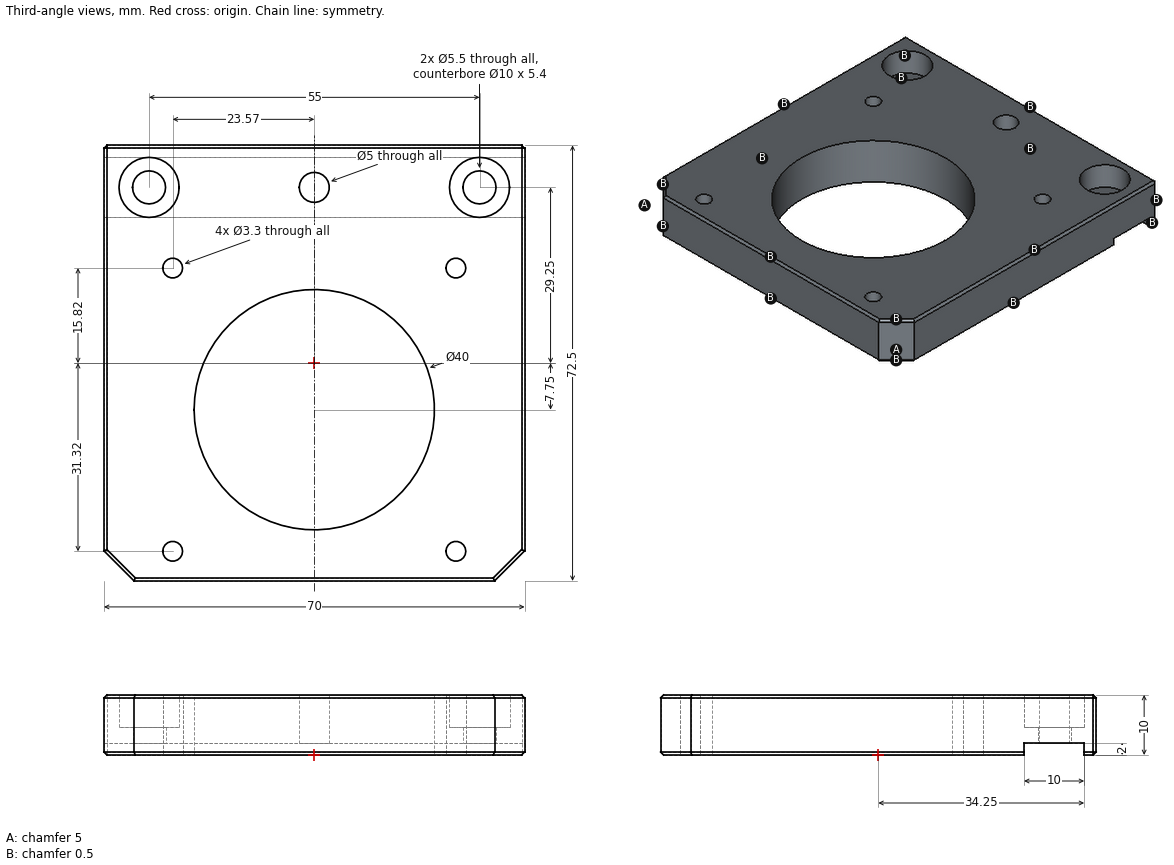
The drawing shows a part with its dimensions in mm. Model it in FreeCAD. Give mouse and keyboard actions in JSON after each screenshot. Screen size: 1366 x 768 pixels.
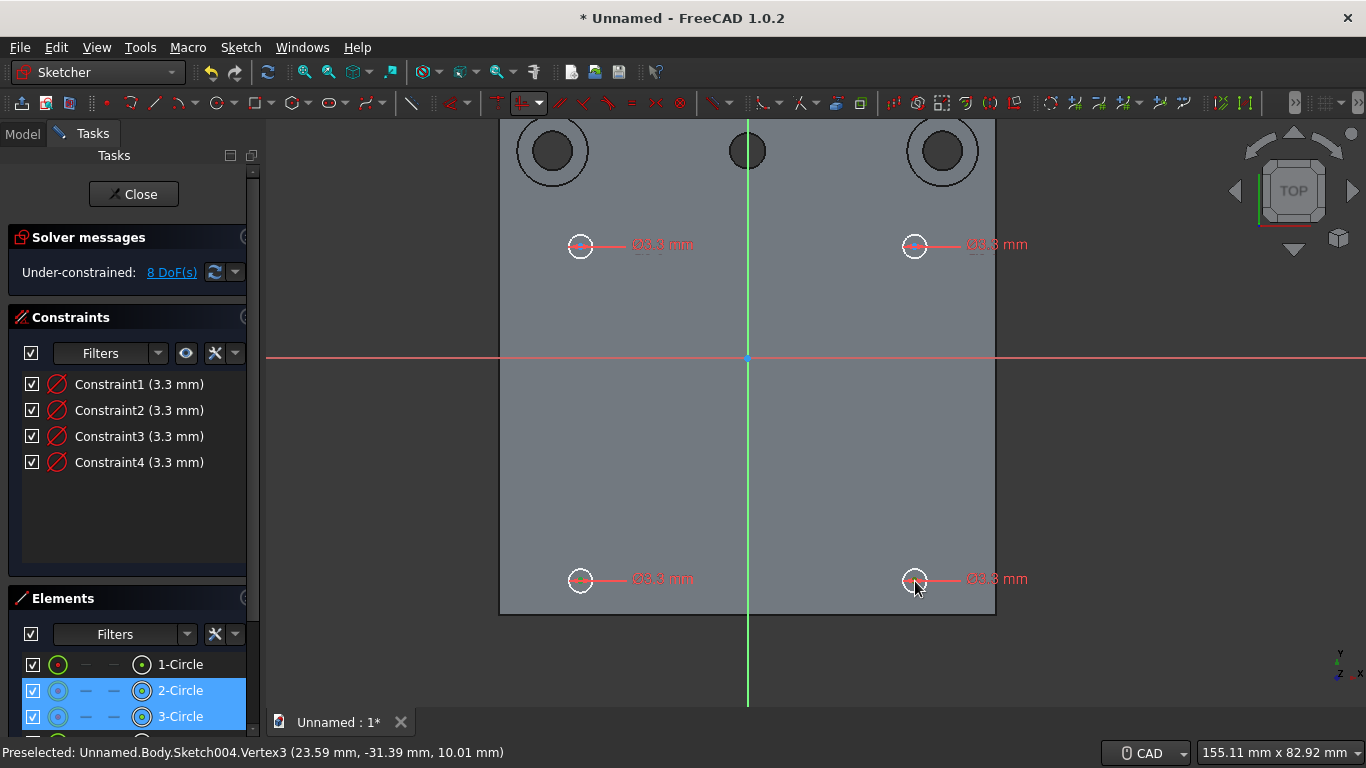
{"action": "left_click", "coordinate": [748, 641]}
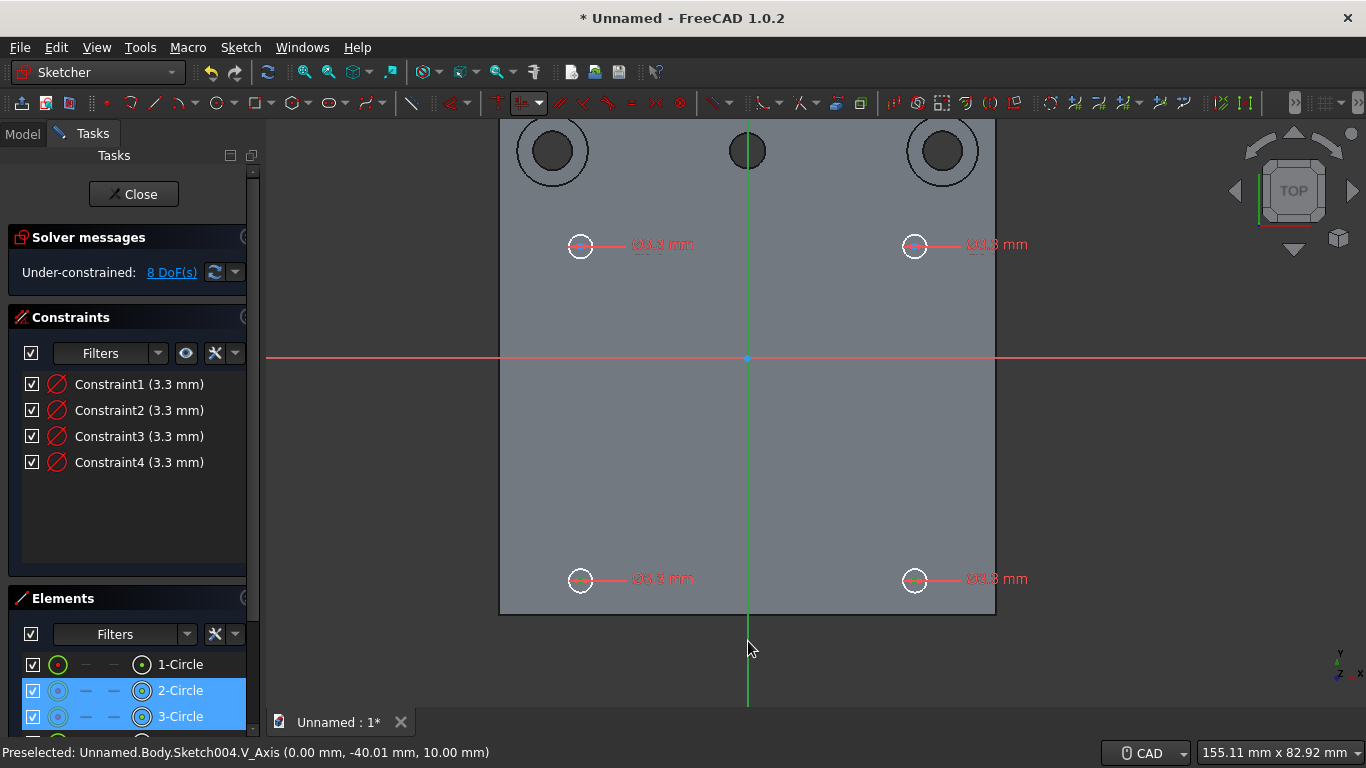
{"action": "left_click", "coordinate": [656, 104]}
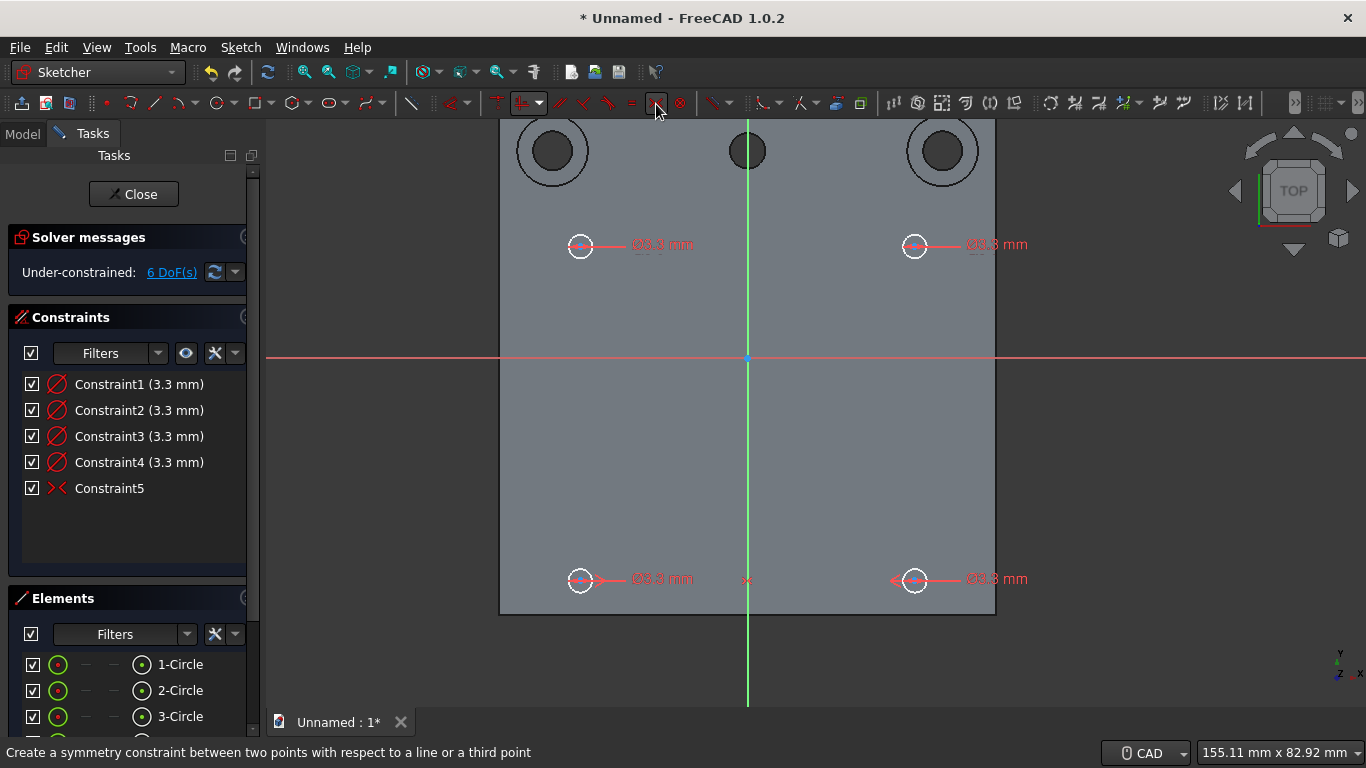
{"action": "left_click", "coordinate": [581, 247]}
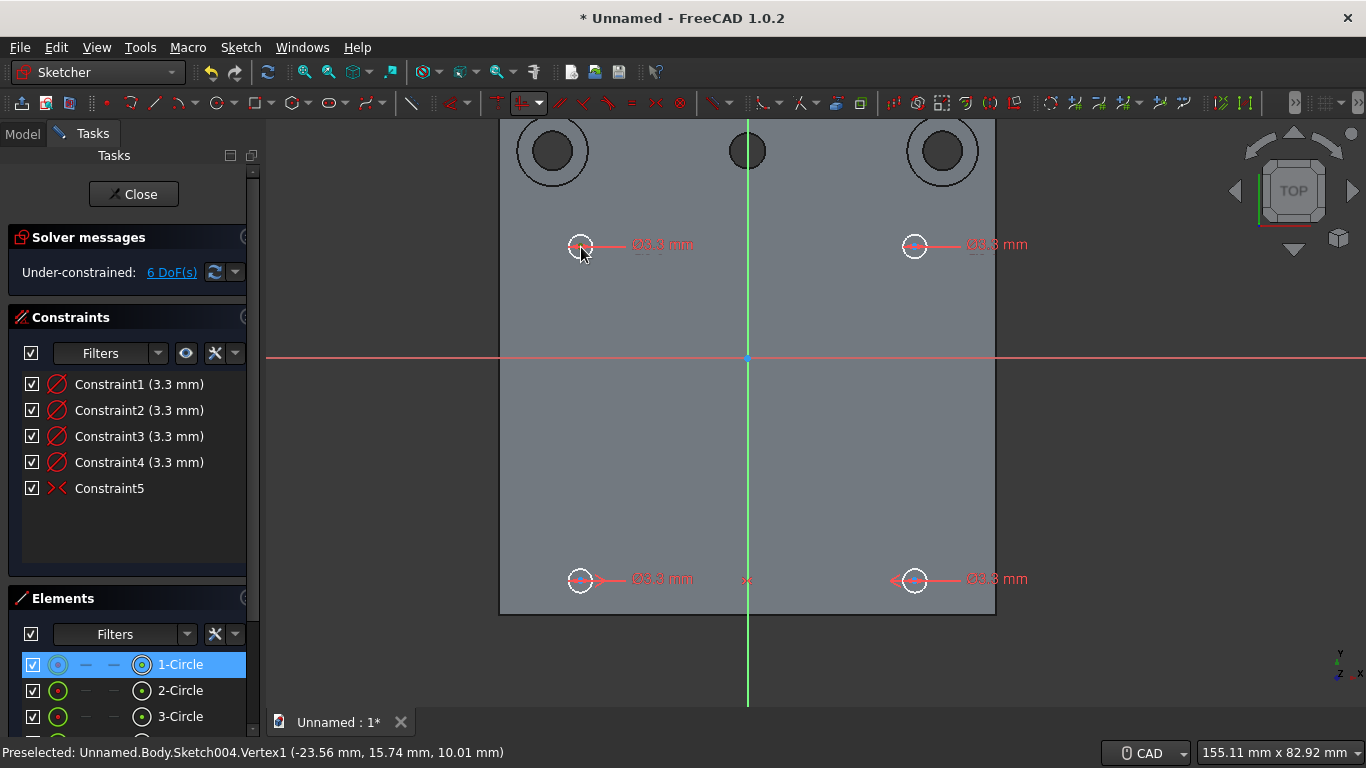
{"action": "left_click", "coordinate": [915, 247]}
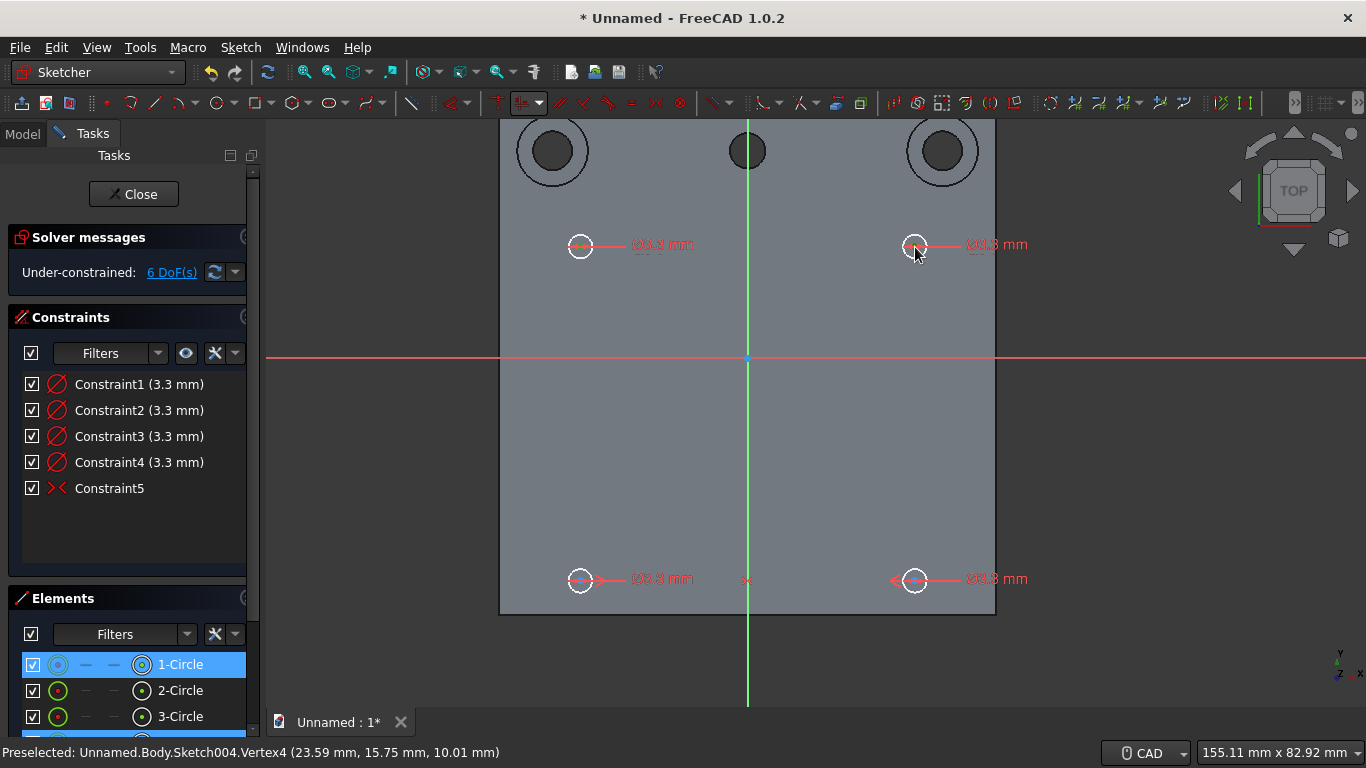
{"action": "left_click", "coordinate": [748, 641]}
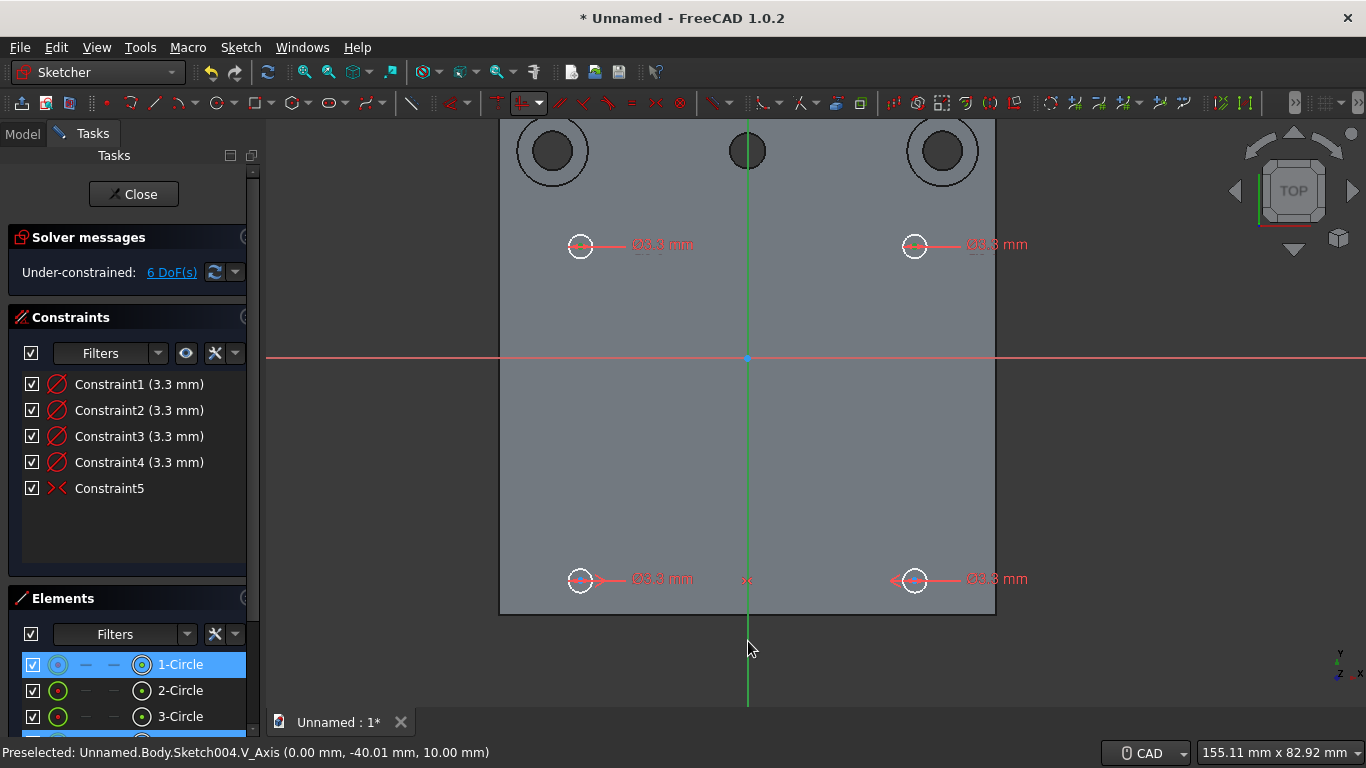
{"action": "left_click", "coordinate": [656, 104]}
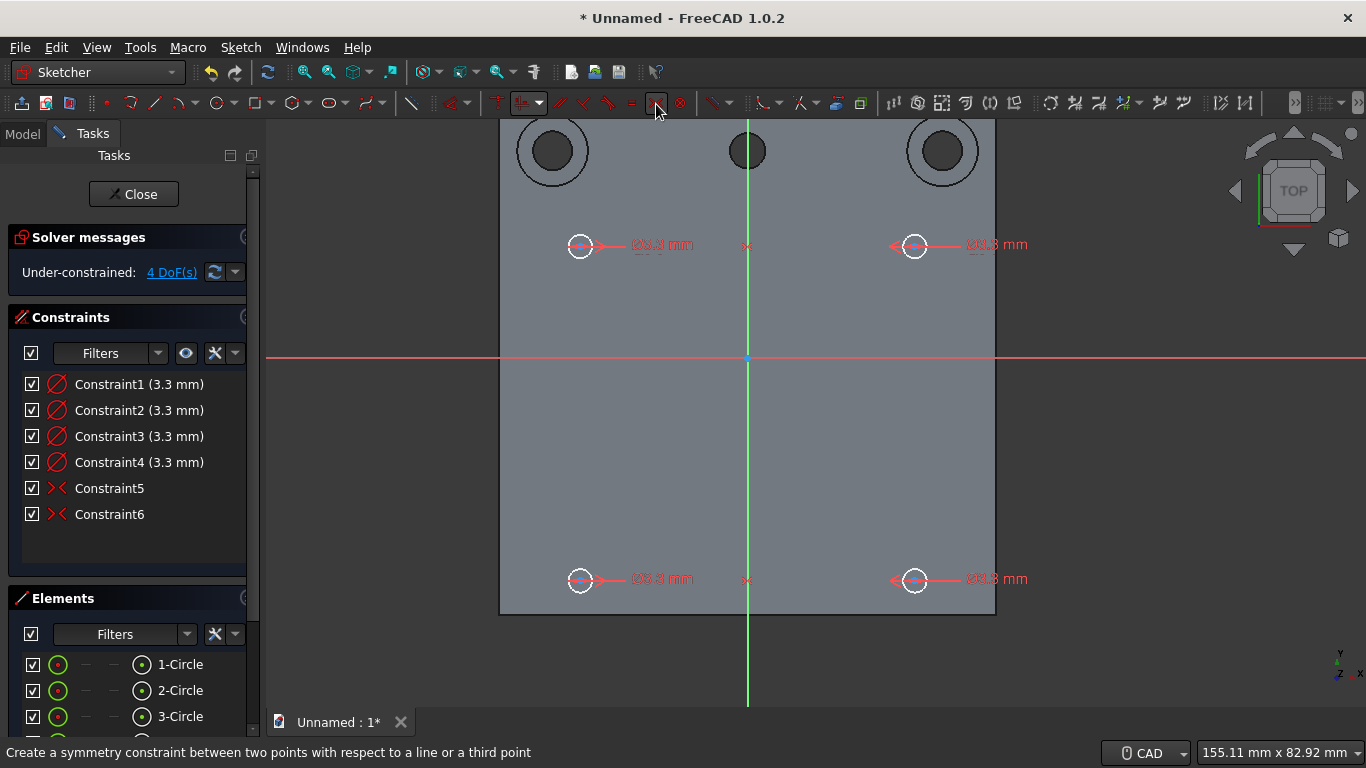
{"action": "left_click", "coordinate": [450, 104]}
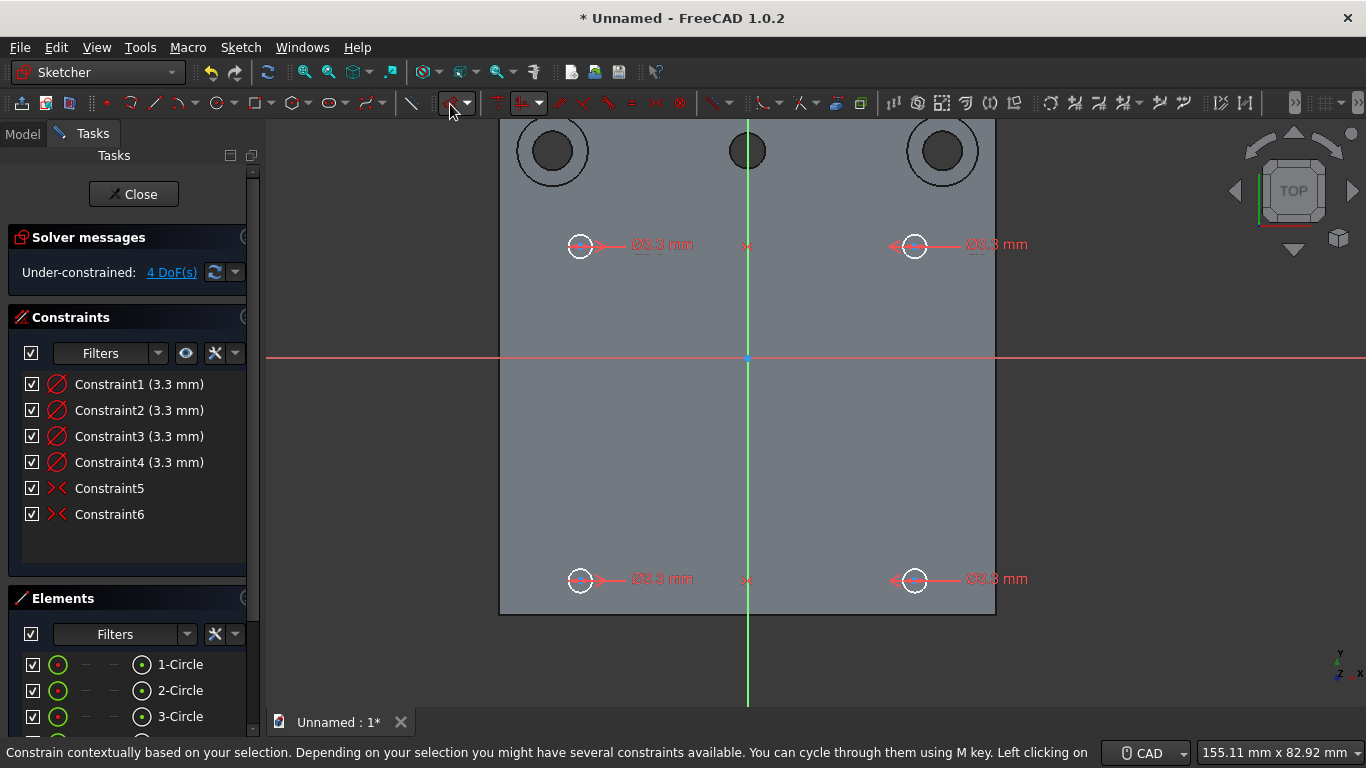
{"action": "left_click", "coordinate": [580, 247]}
{"action": "left_click", "coordinate": [664, 213]}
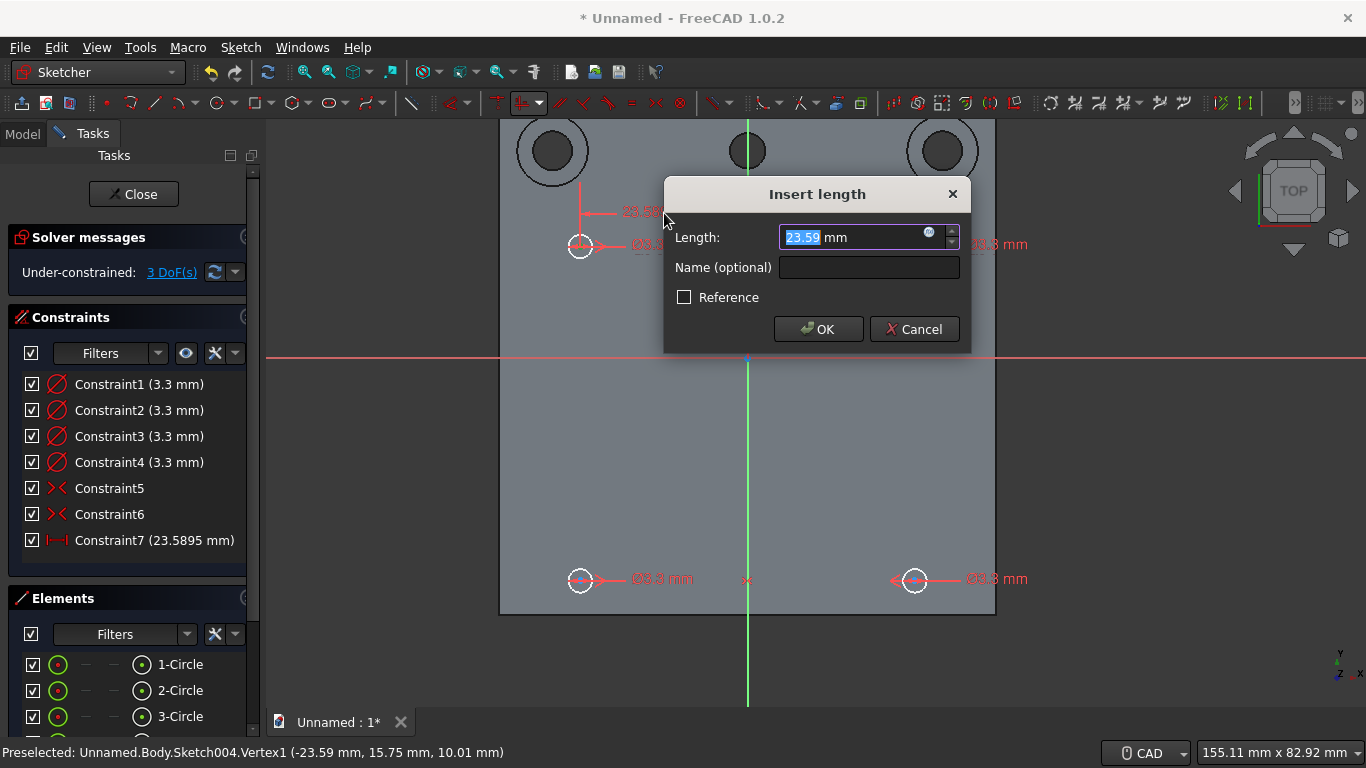
{"action": "type", "text": "23.57"}
{"action": "key", "text": "Return"}